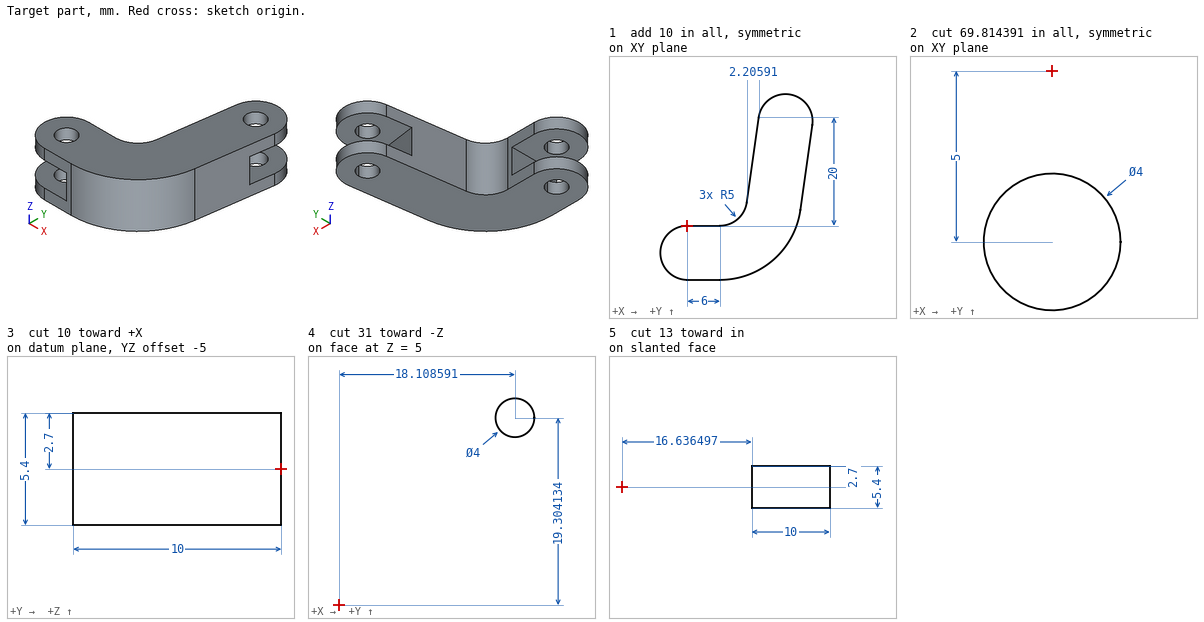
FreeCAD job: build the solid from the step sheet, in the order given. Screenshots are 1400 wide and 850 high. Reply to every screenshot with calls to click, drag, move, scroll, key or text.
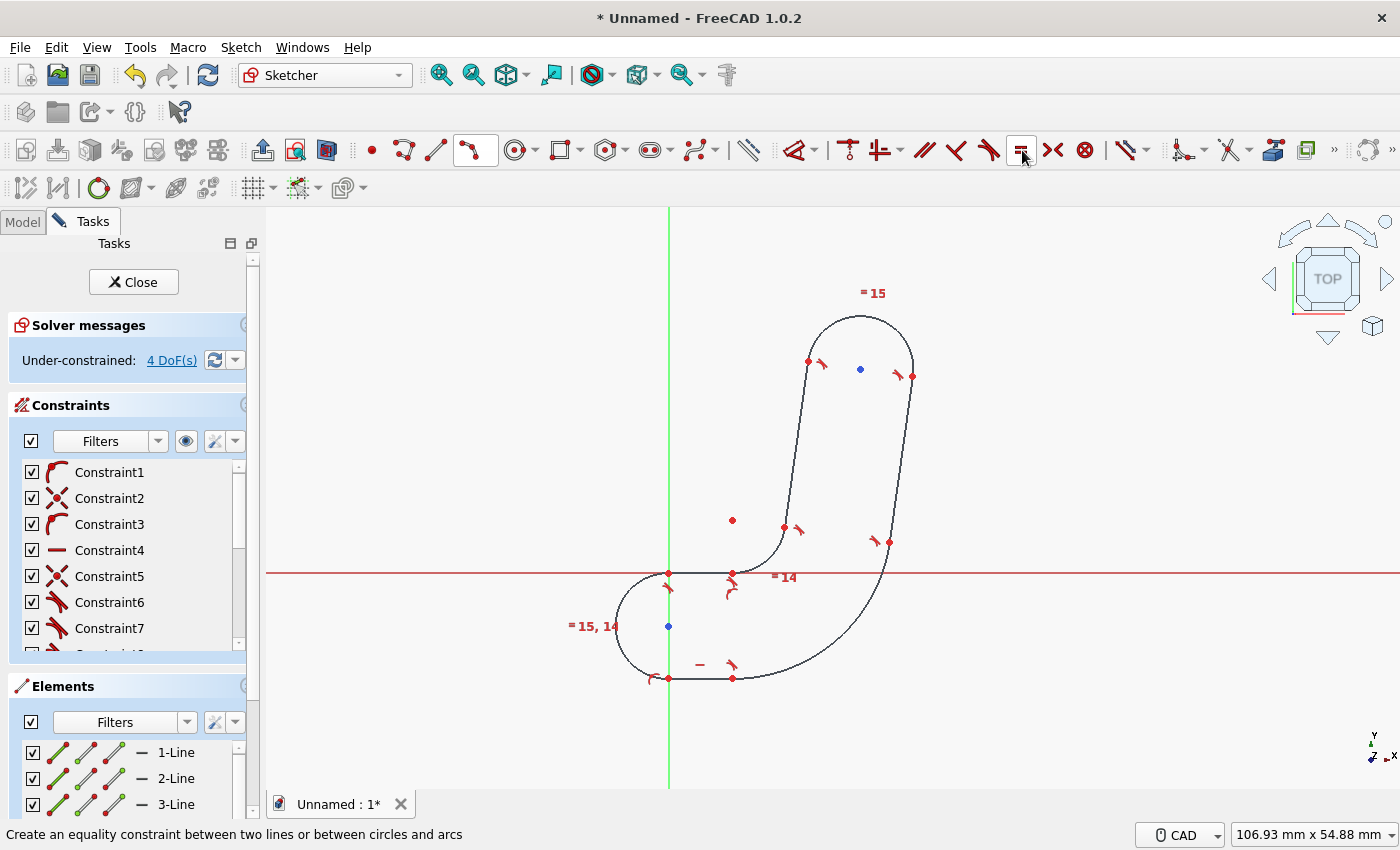
click(777, 549)
click(773, 595)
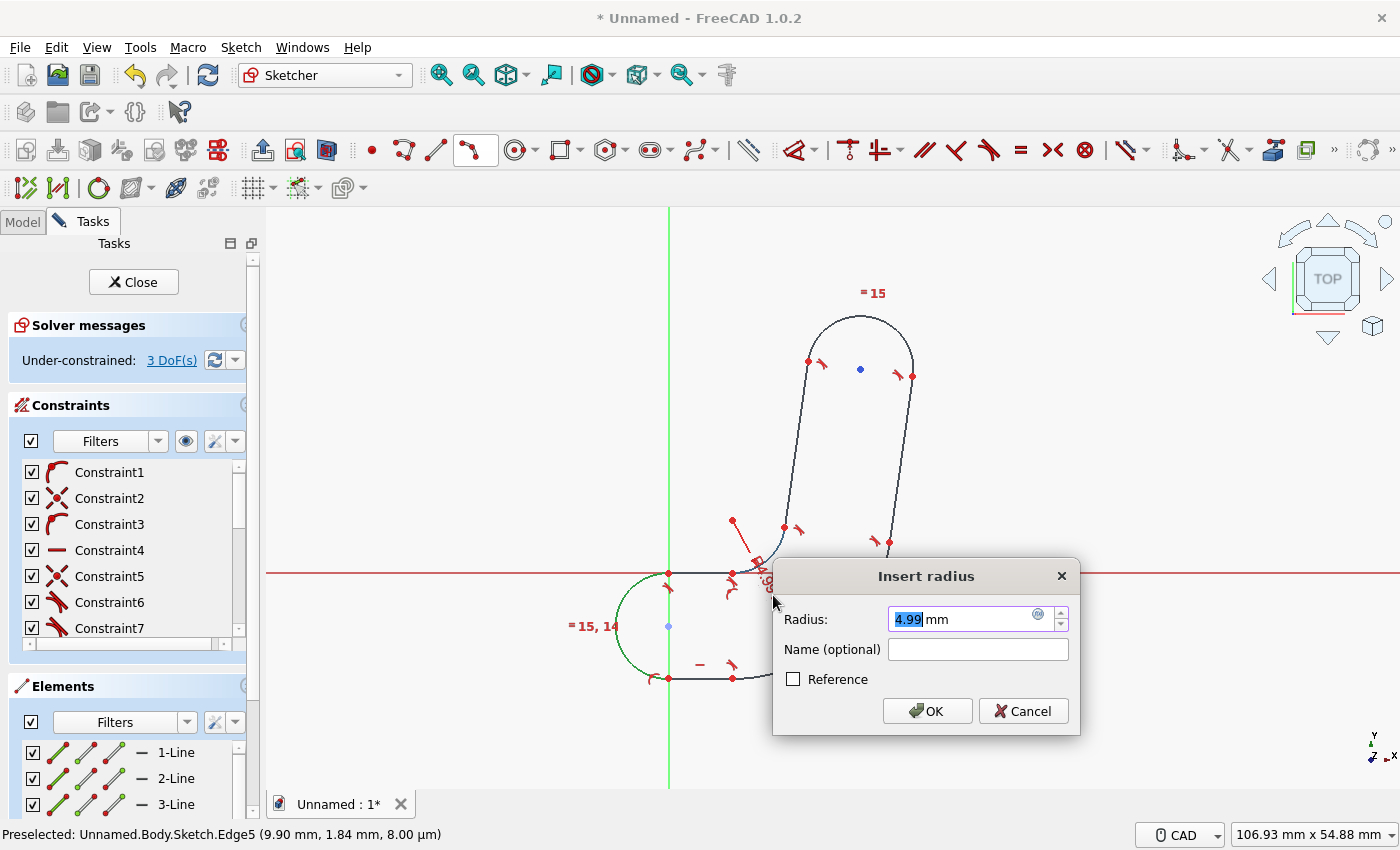
text(5)
key(Return)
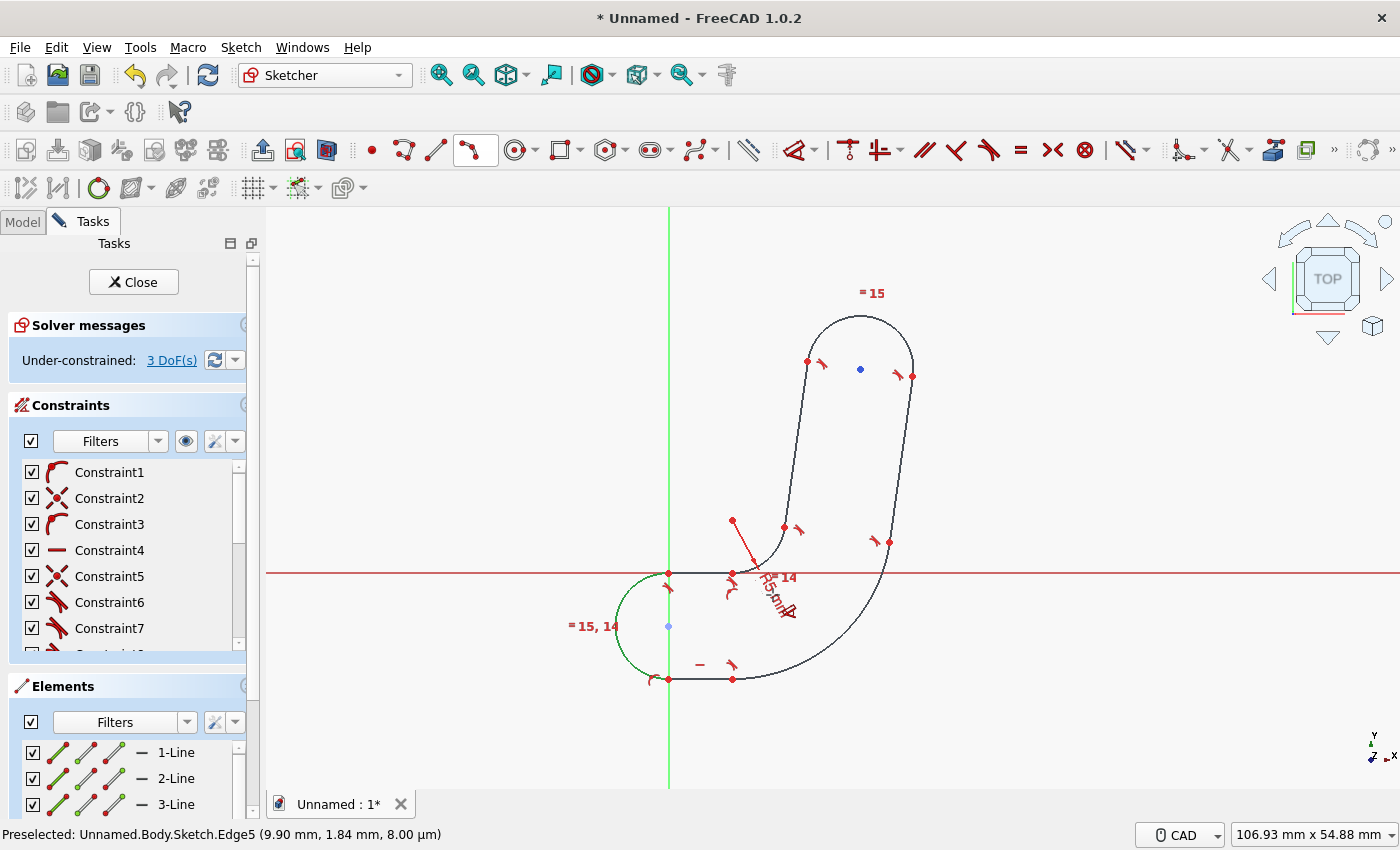
click(713, 573)
click(700, 607)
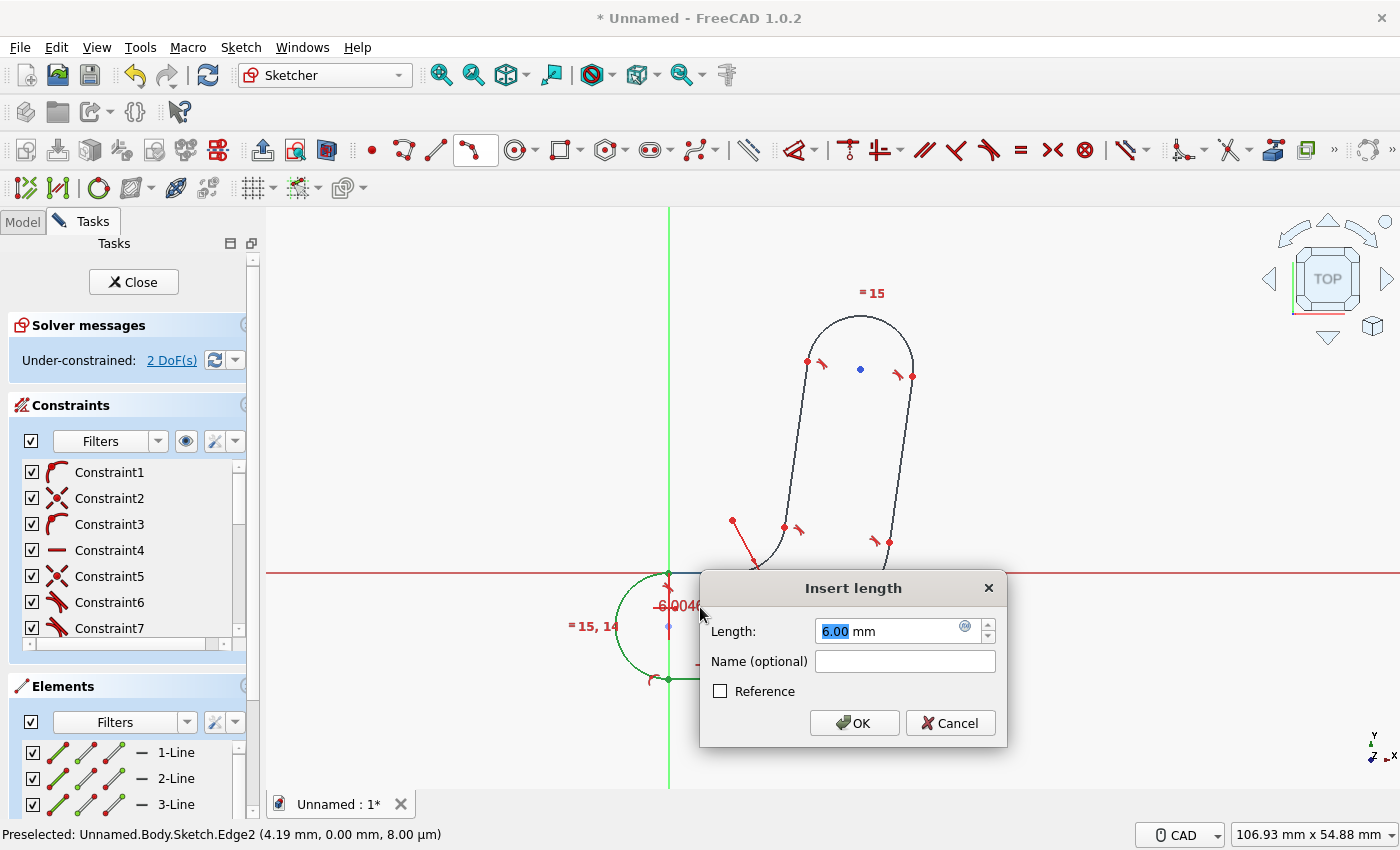
text(6)
key(Return)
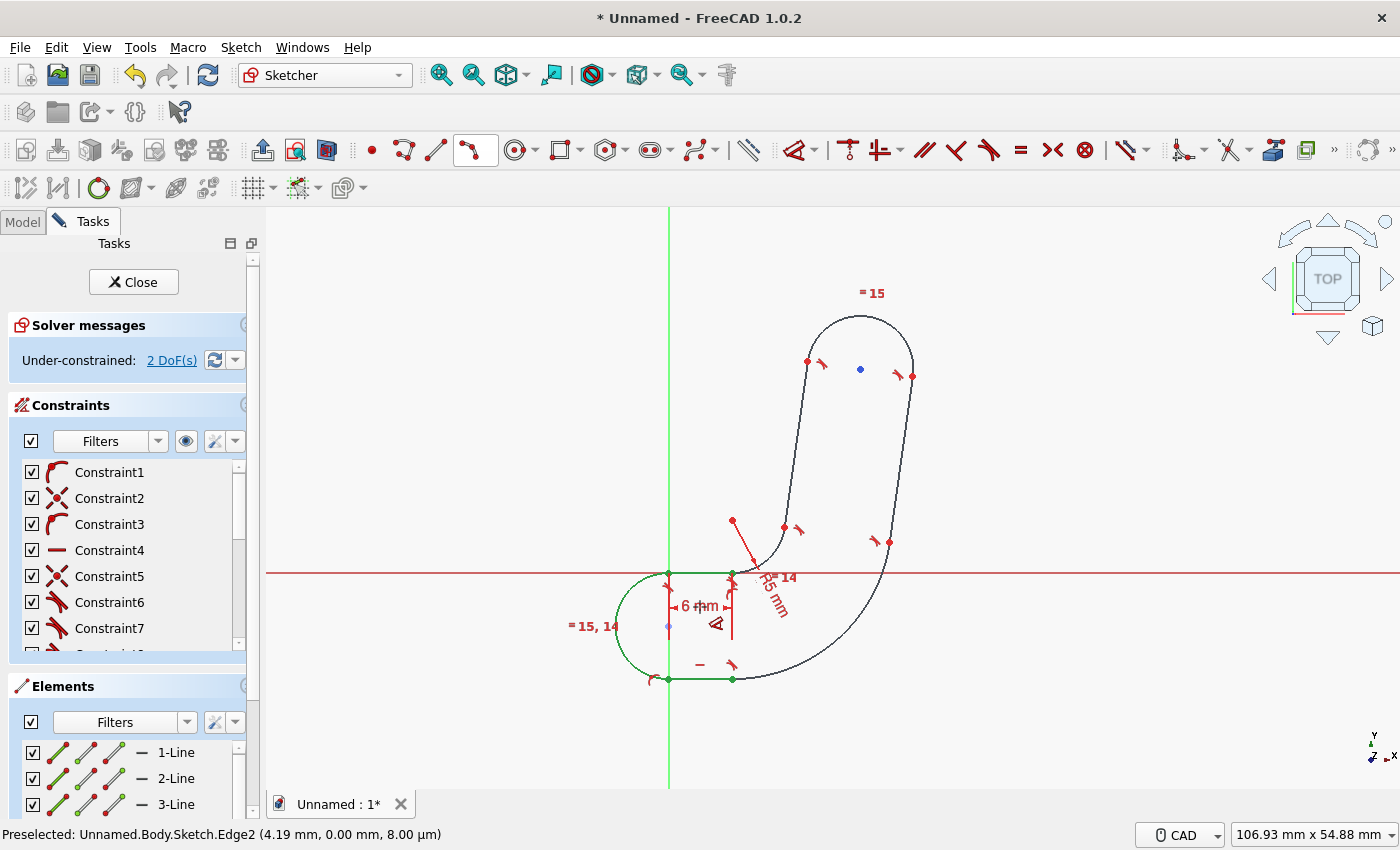
click(808, 362)
click(635, 467)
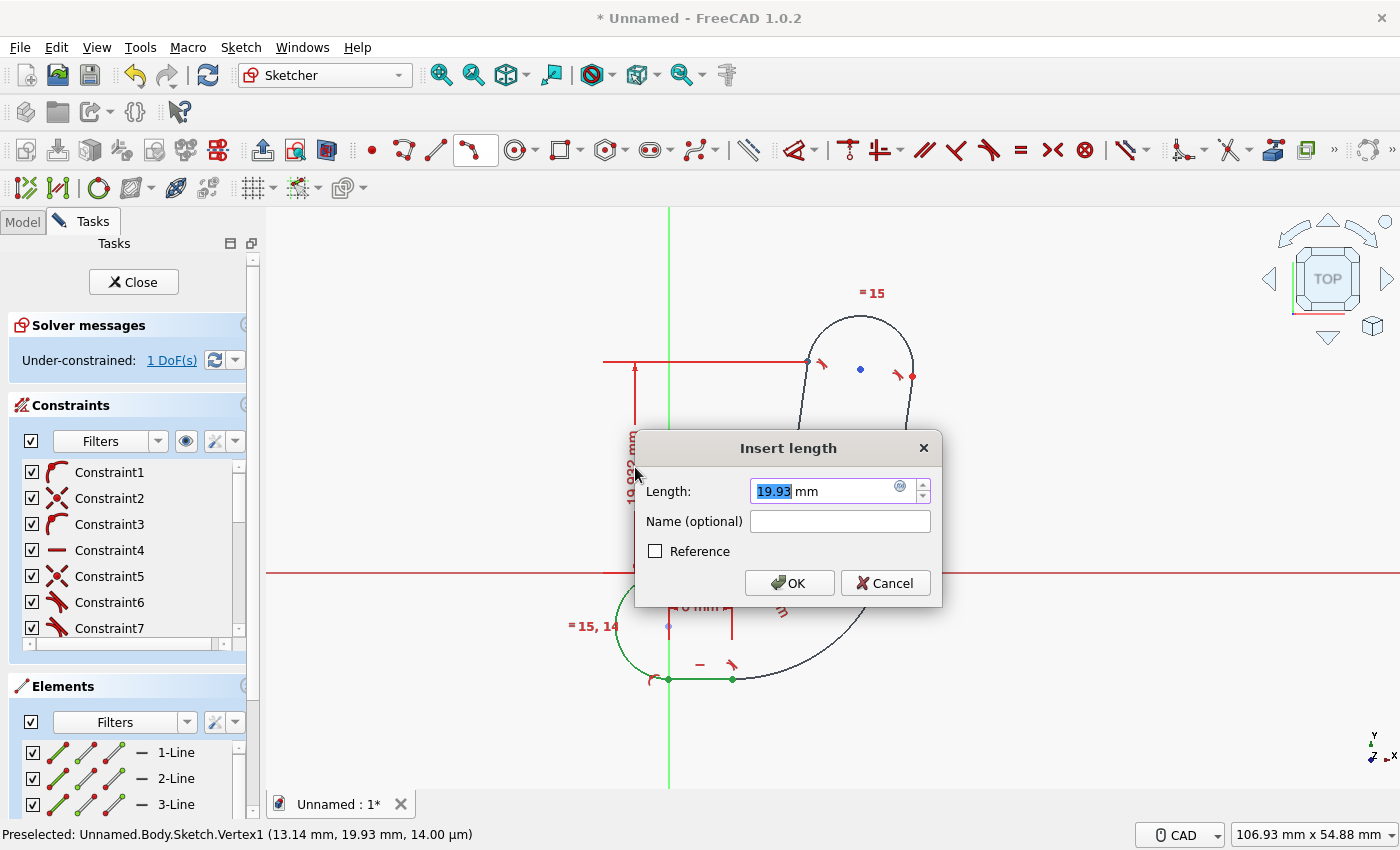
text(20)
key(Return)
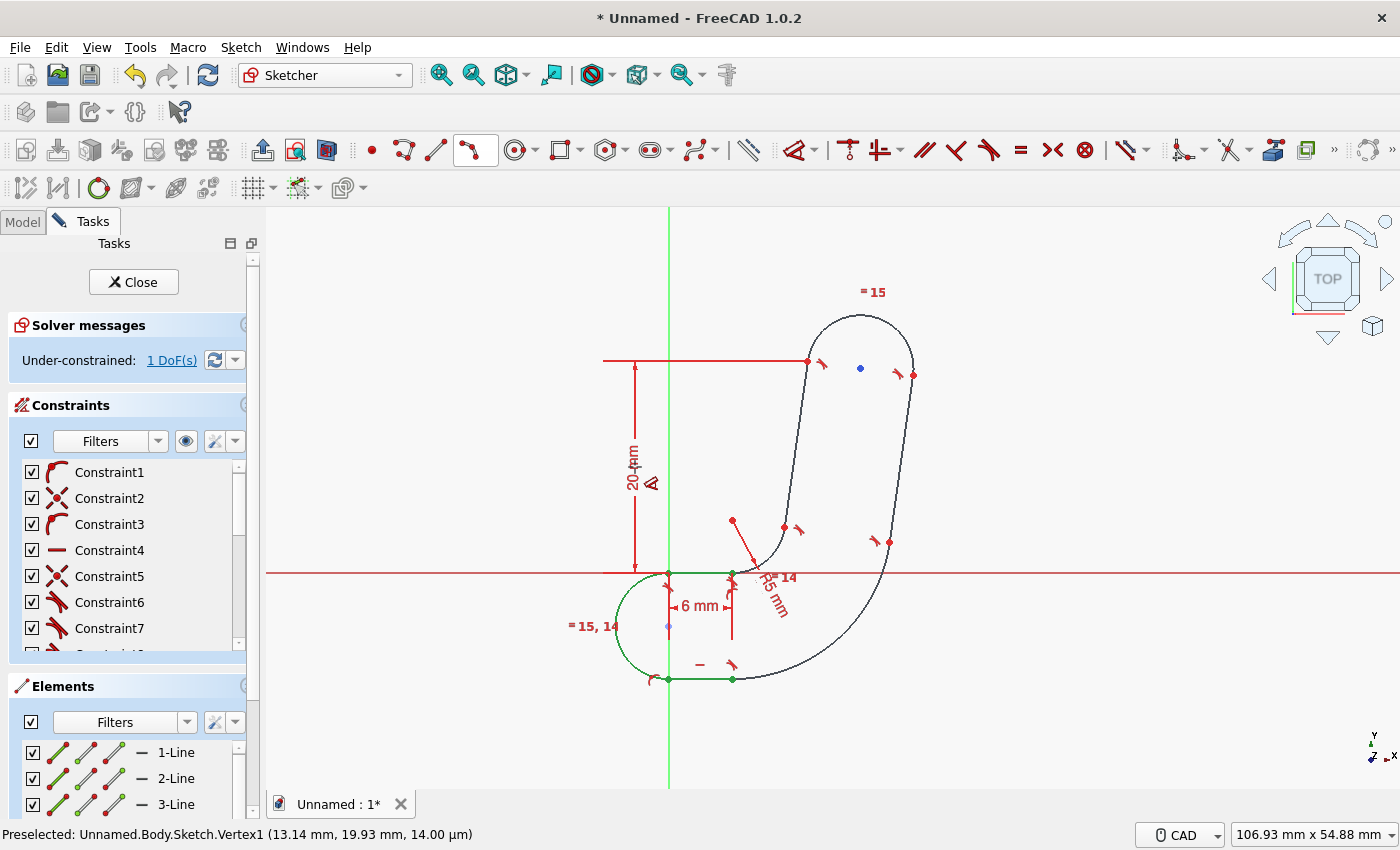
scroll(801, 411, up, 3)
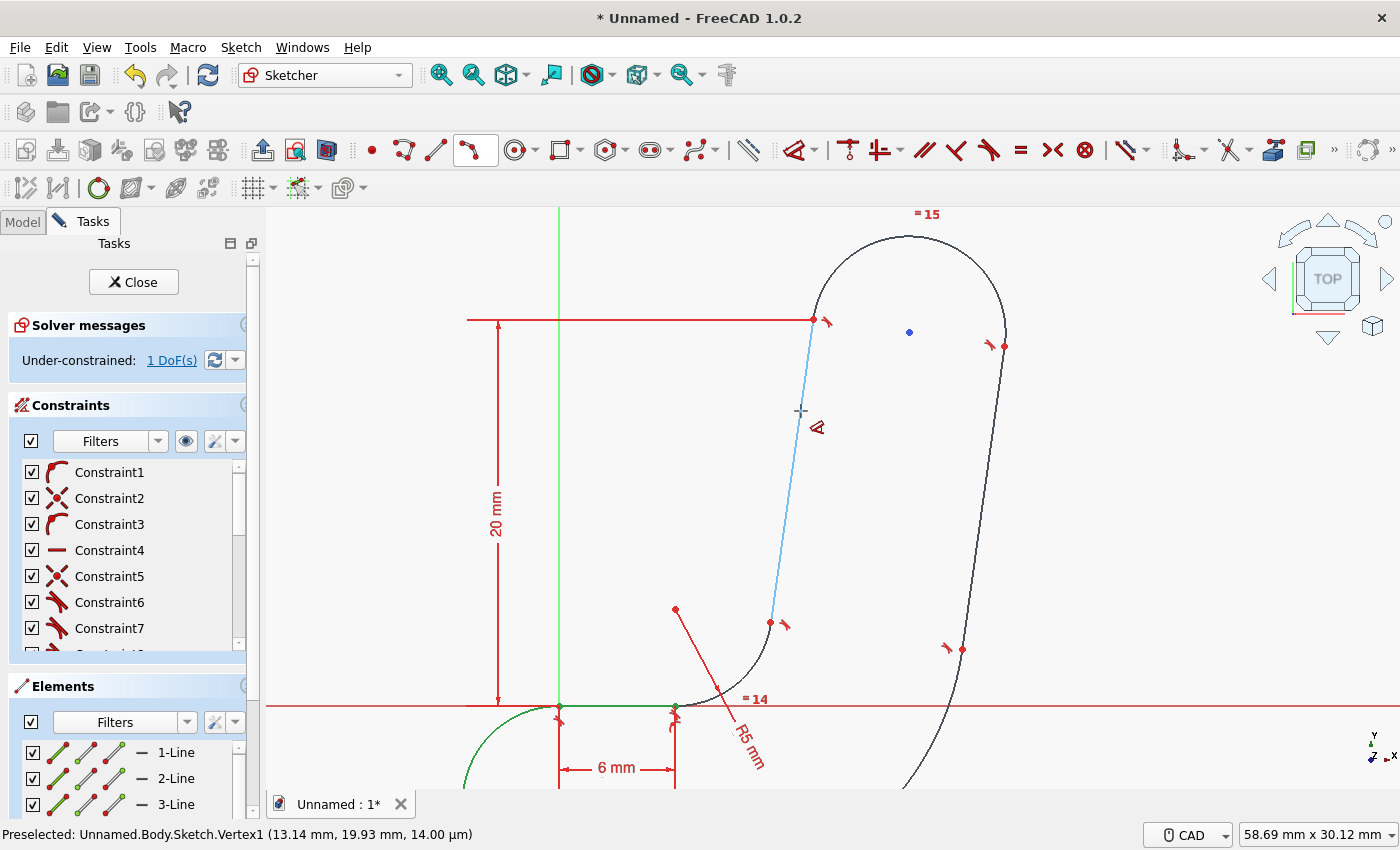
click(801, 411)
click(792, 286)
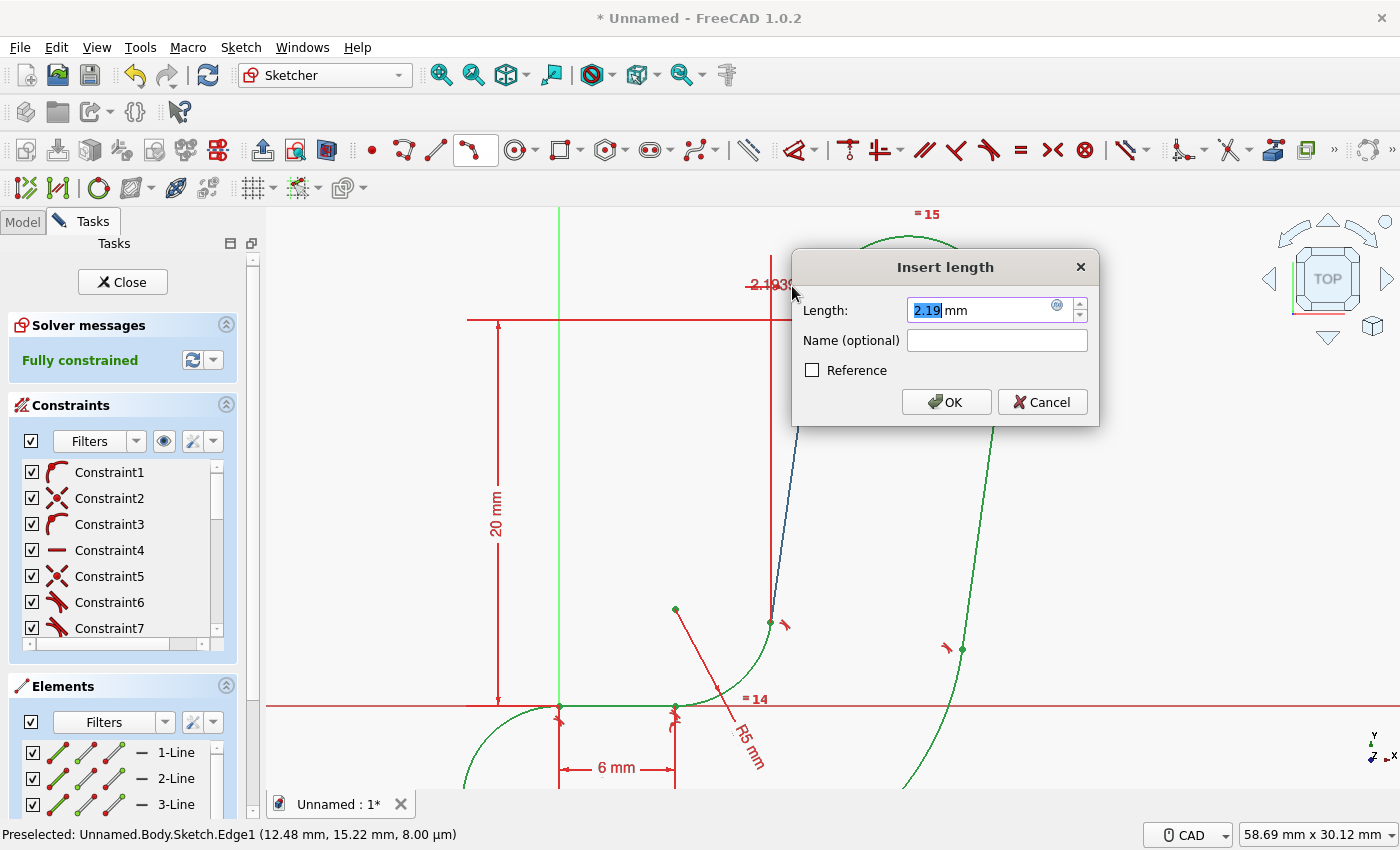
text(2.20591)
key(Return)
key(Escape)